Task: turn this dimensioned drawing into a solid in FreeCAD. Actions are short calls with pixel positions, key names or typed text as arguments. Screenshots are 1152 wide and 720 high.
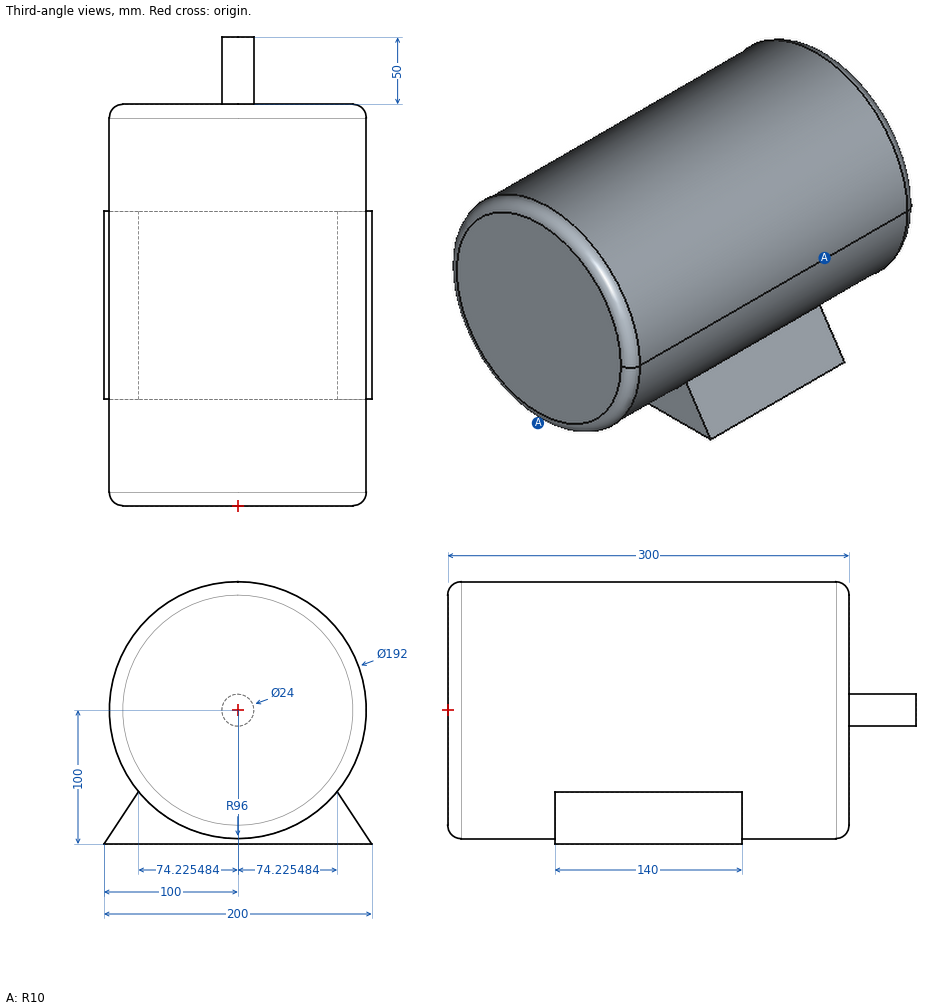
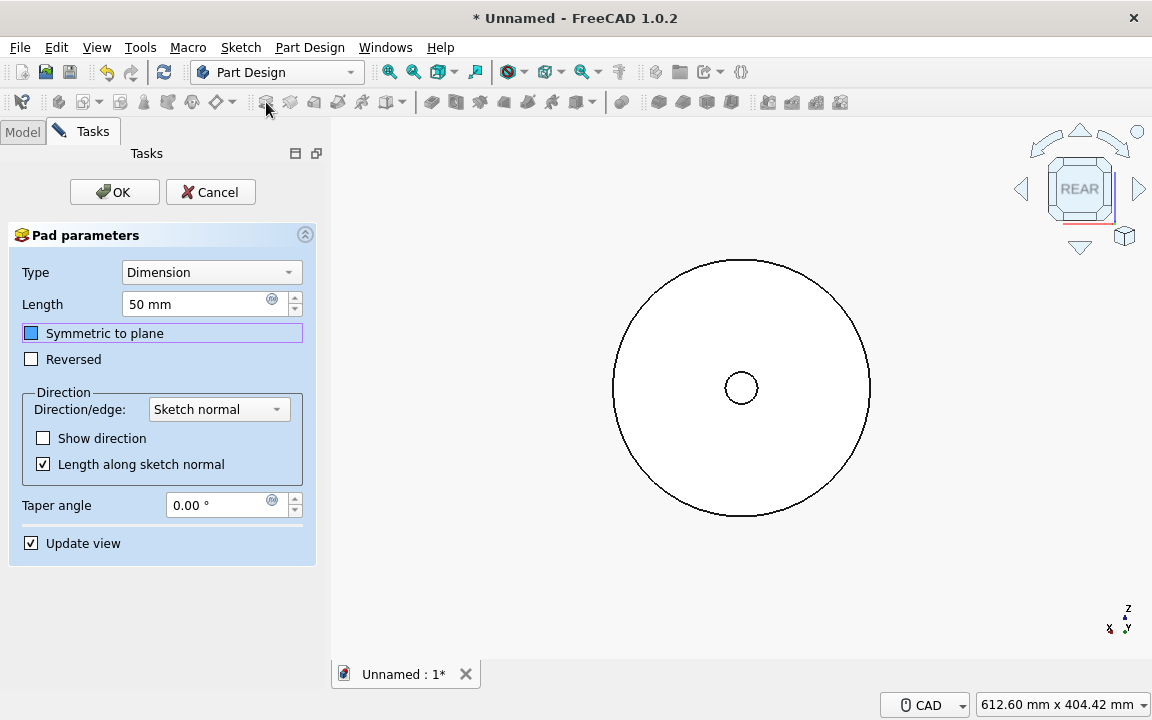
click(115, 192)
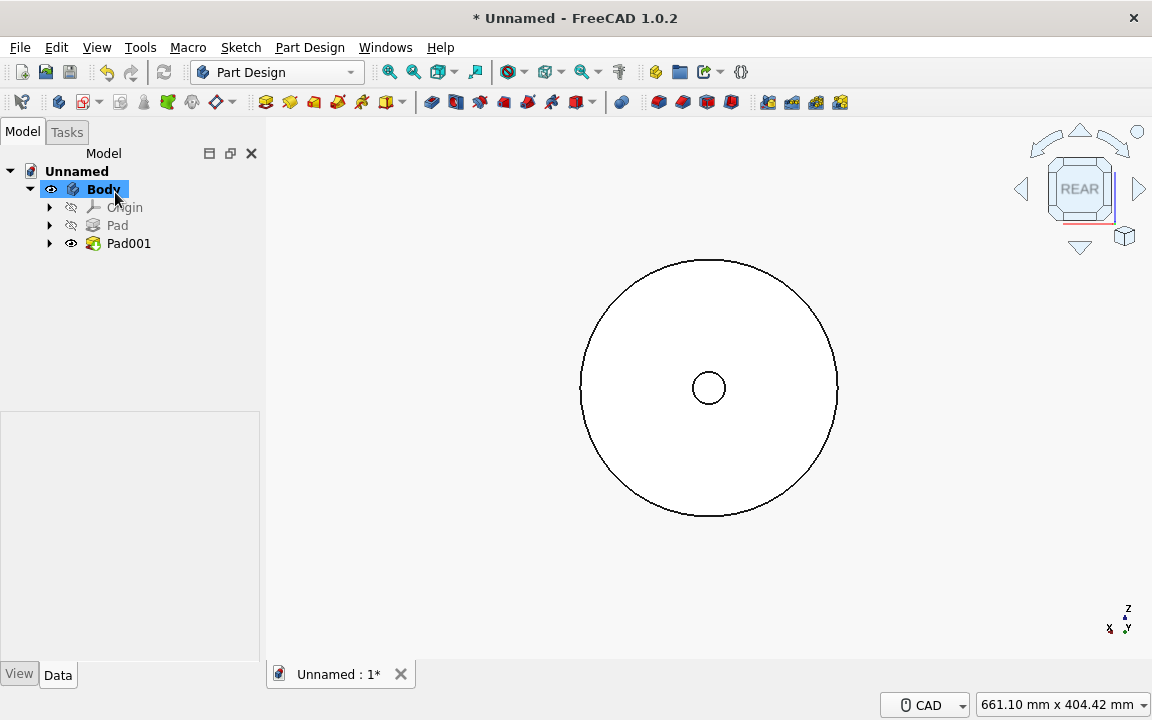
click(838, 387)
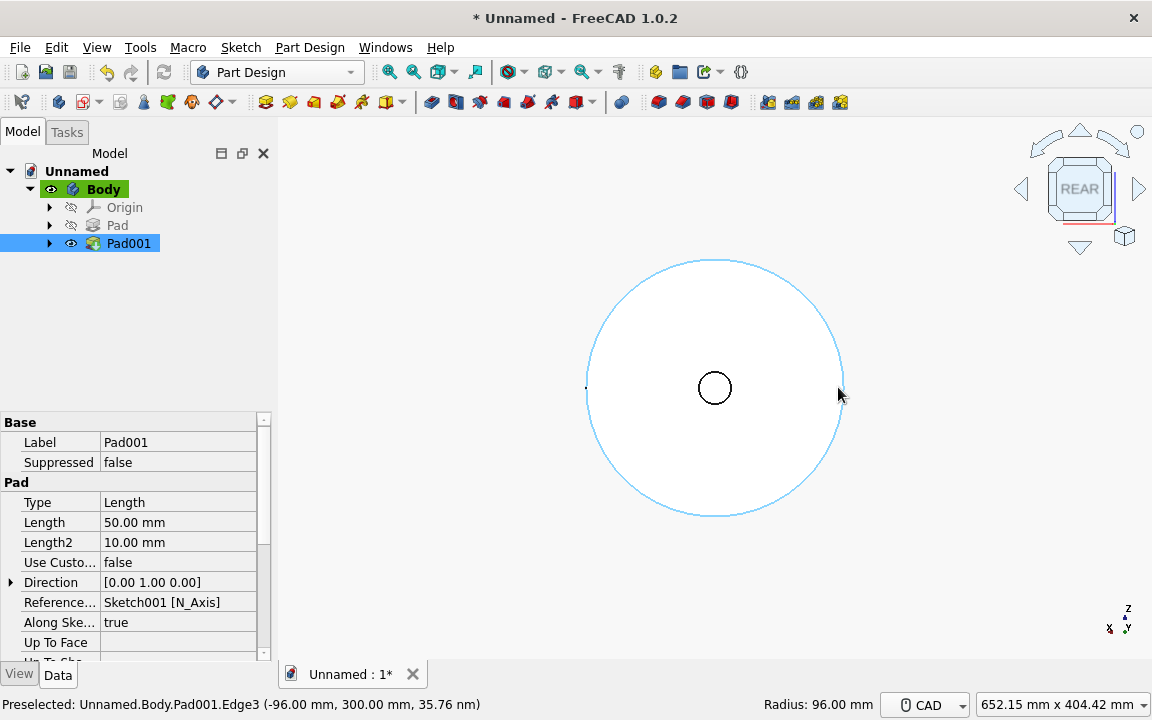
key(0)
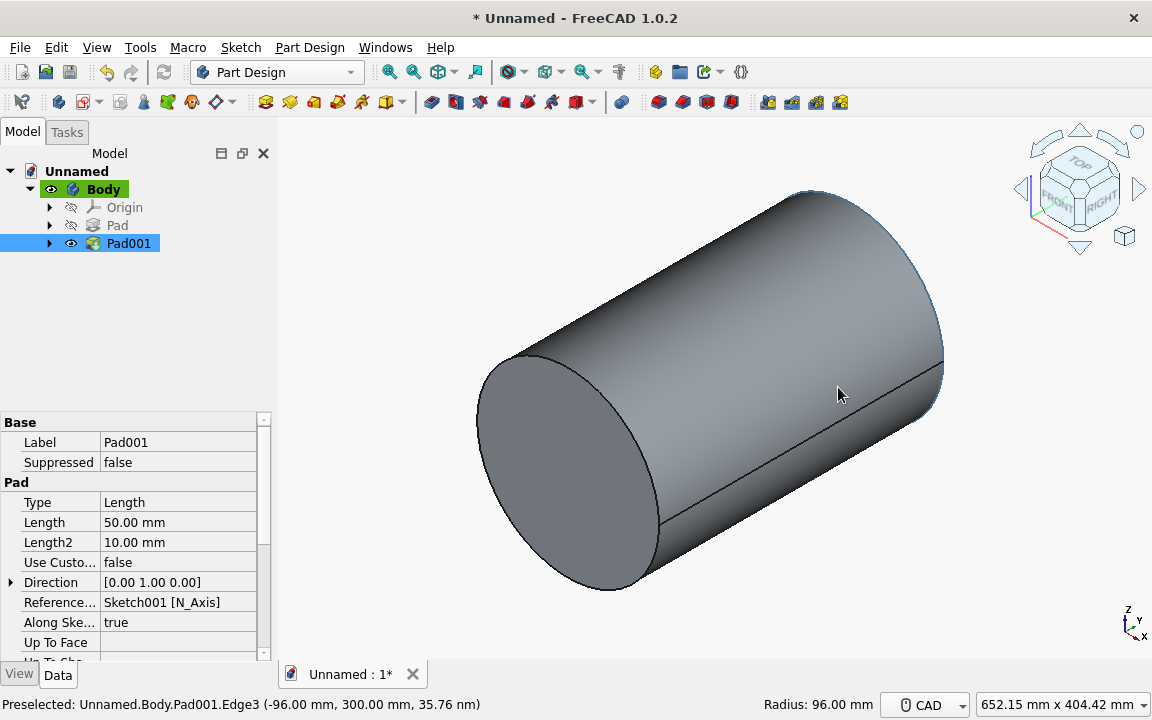
click(540, 356, ctrl)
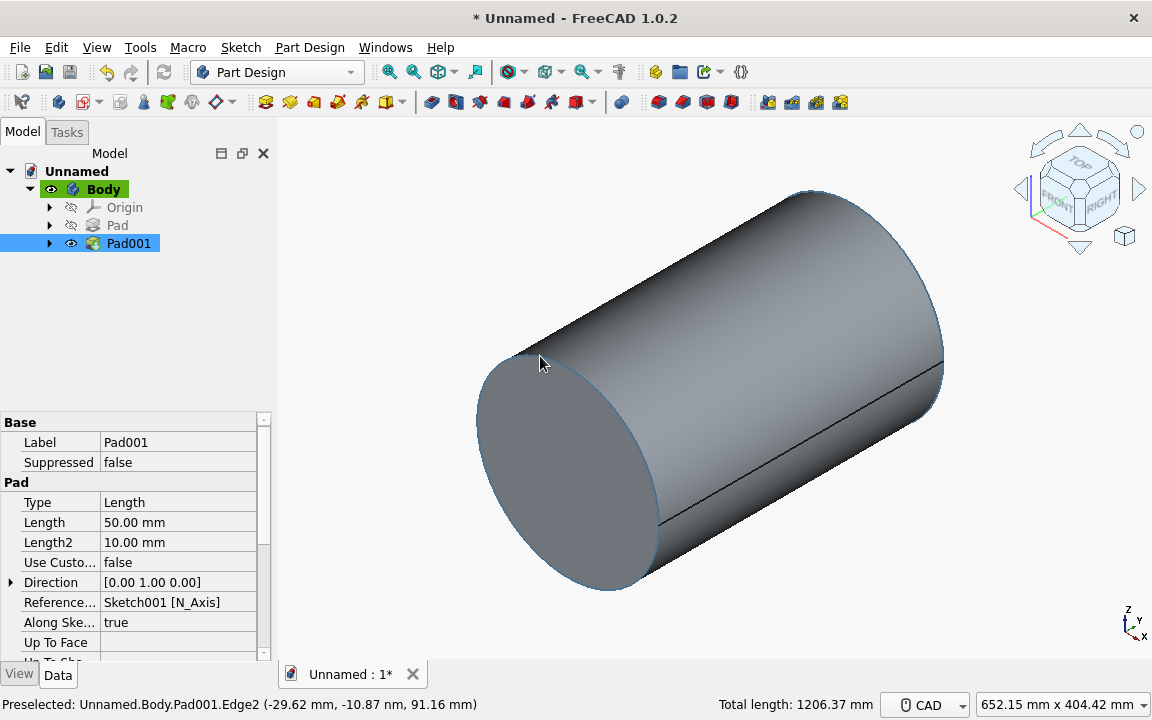
click(660, 102)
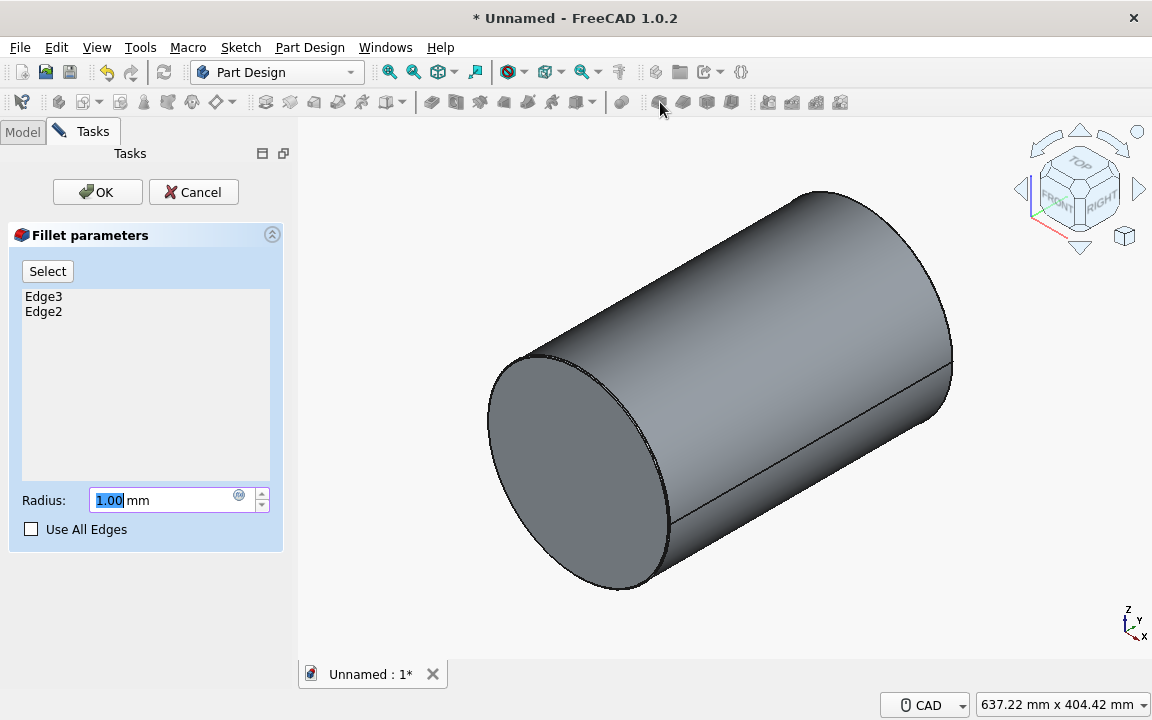
text(10)
key(Tab)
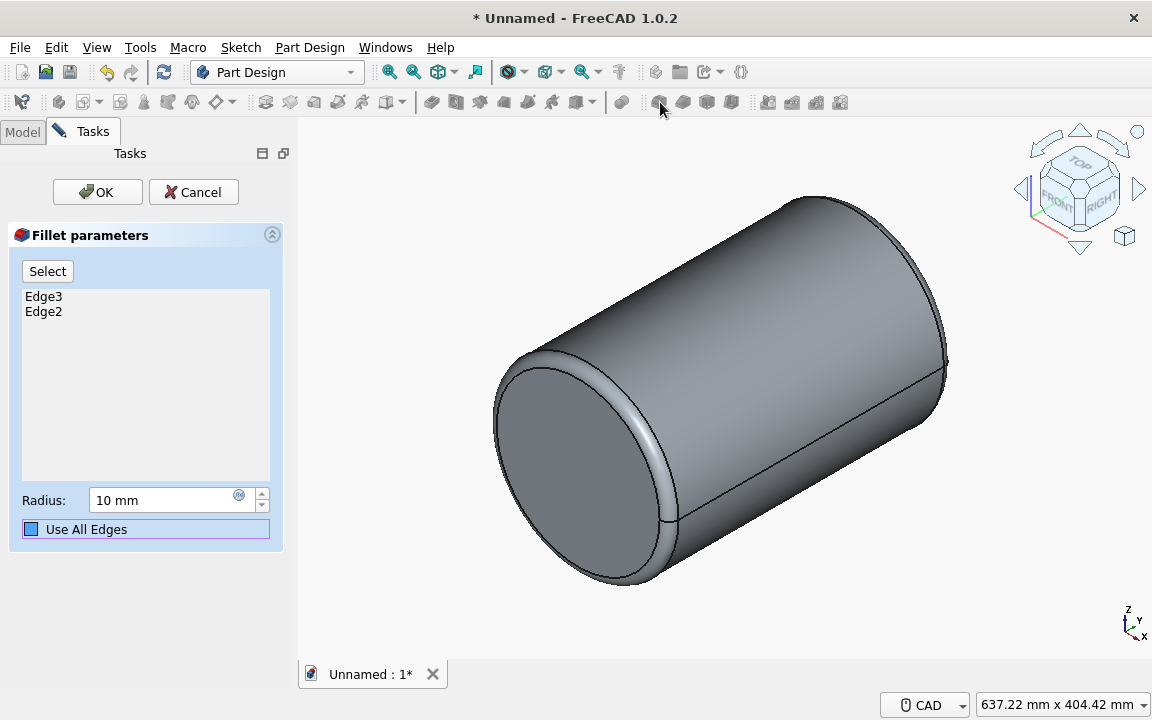
click(98, 192)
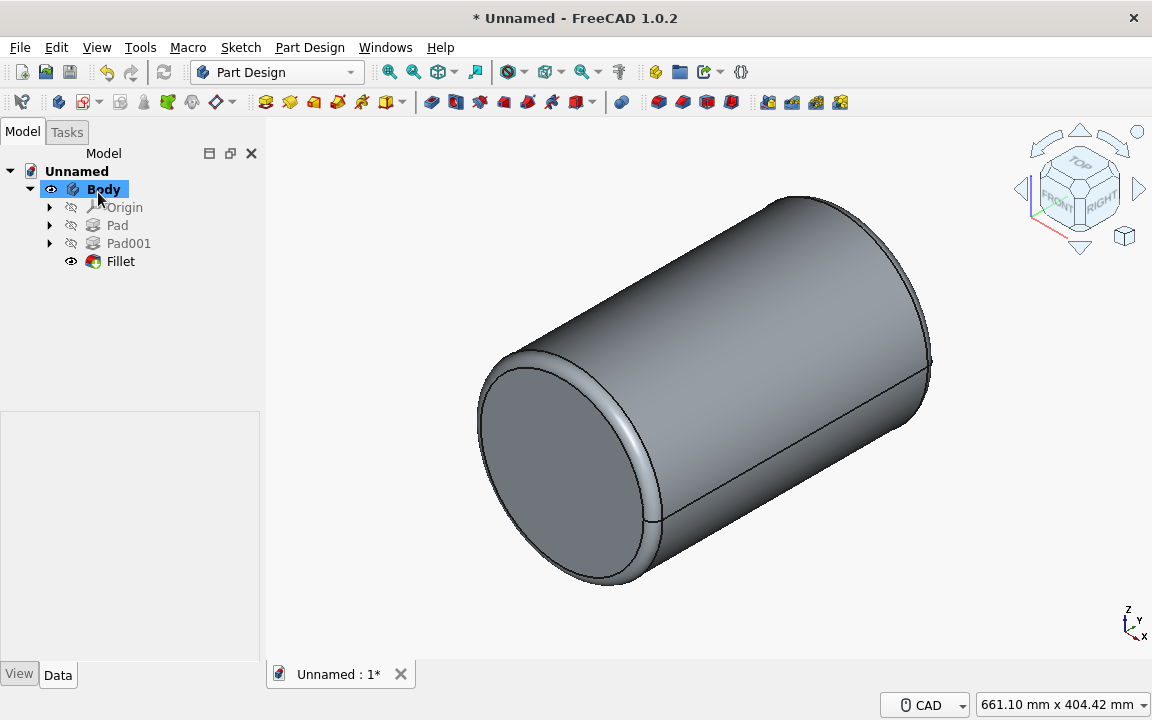
click(50, 207)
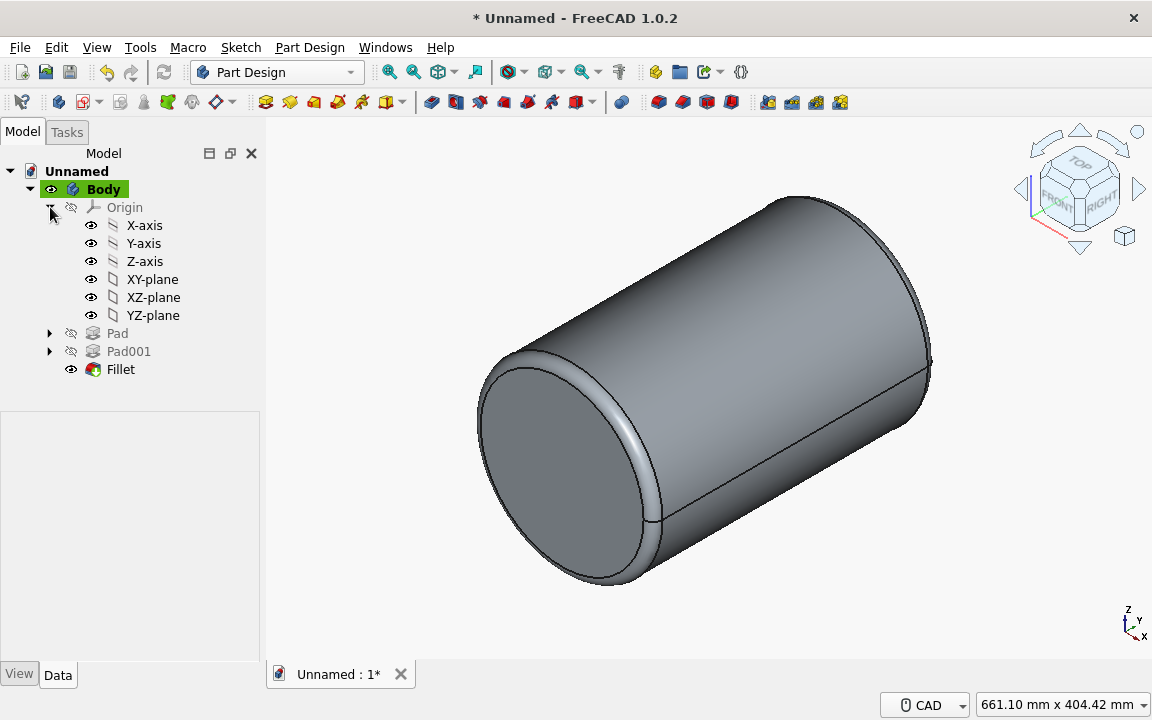
click(136, 297)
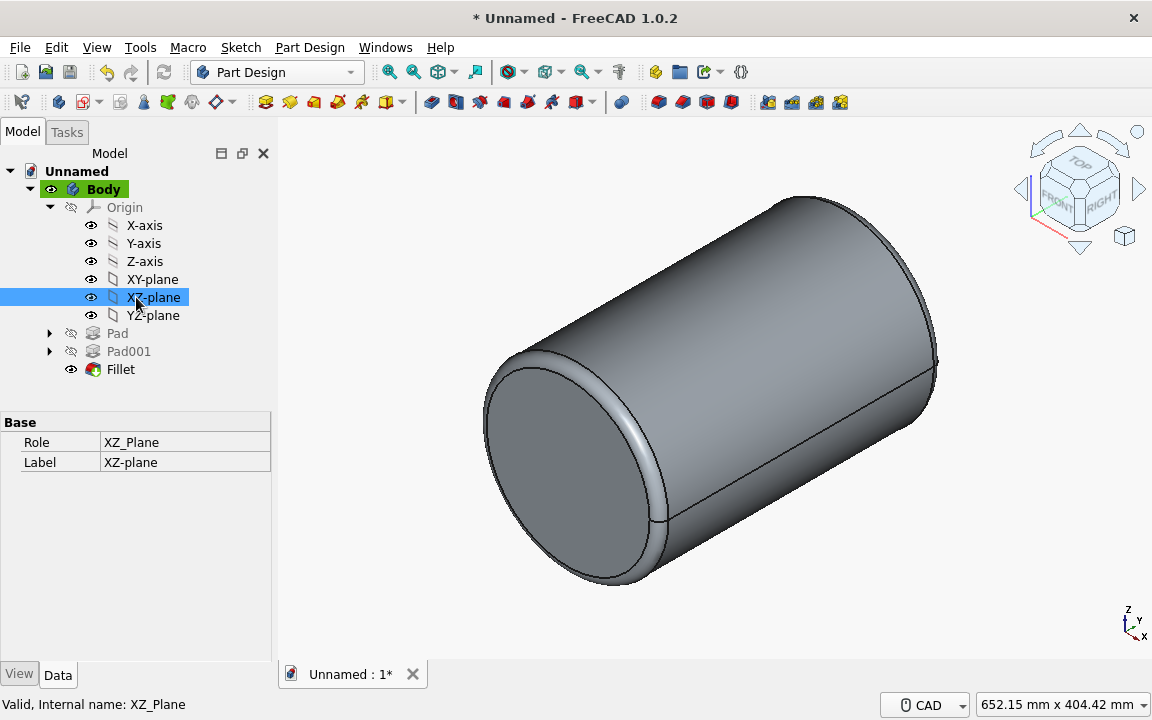
click(216, 102)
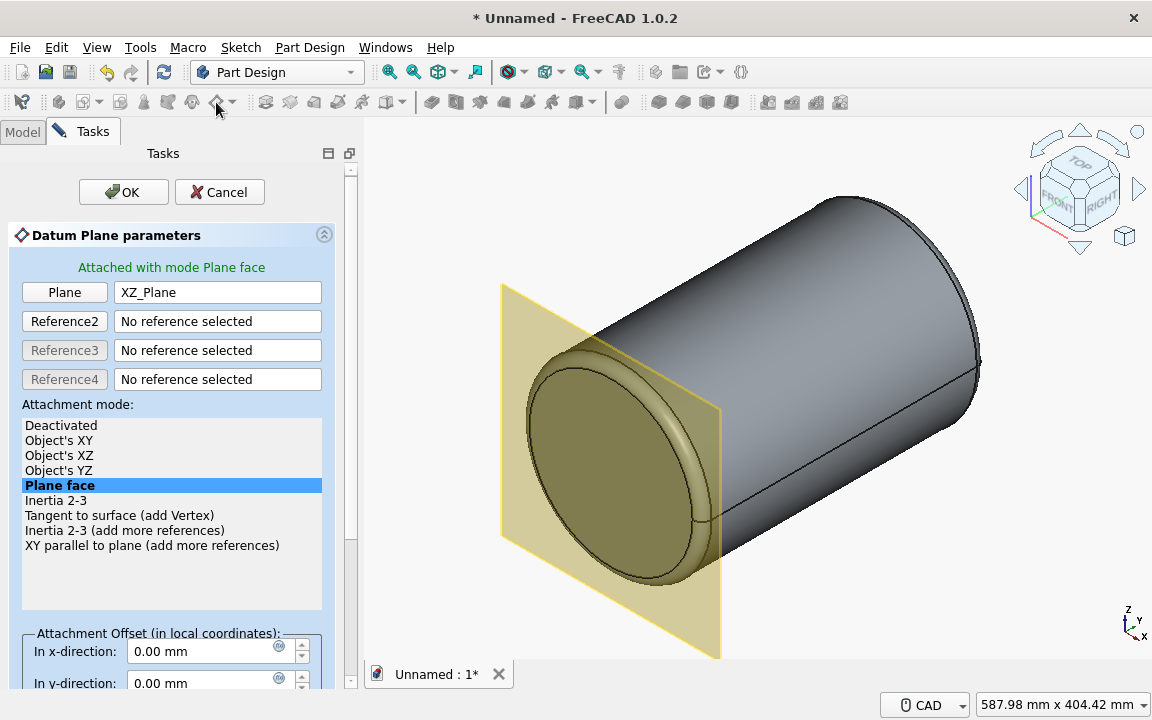
scroll(351, 426, down, 2)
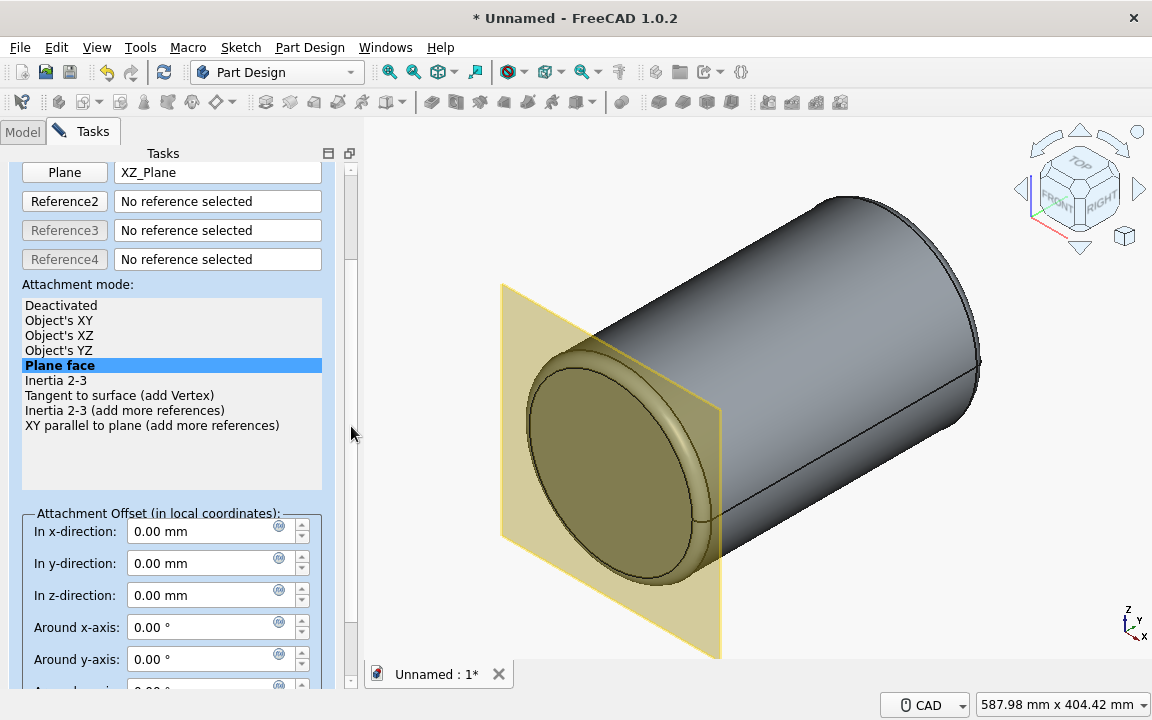
triple_click(210, 595)